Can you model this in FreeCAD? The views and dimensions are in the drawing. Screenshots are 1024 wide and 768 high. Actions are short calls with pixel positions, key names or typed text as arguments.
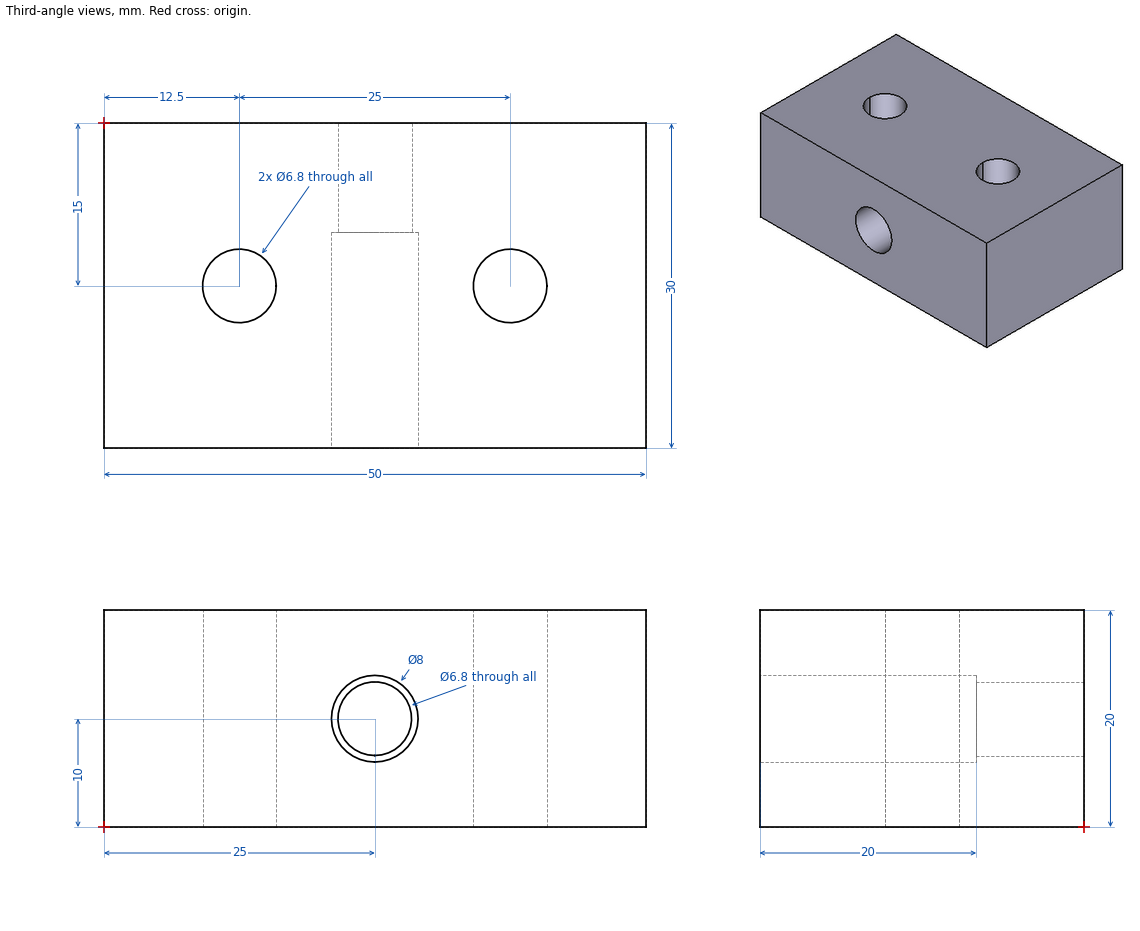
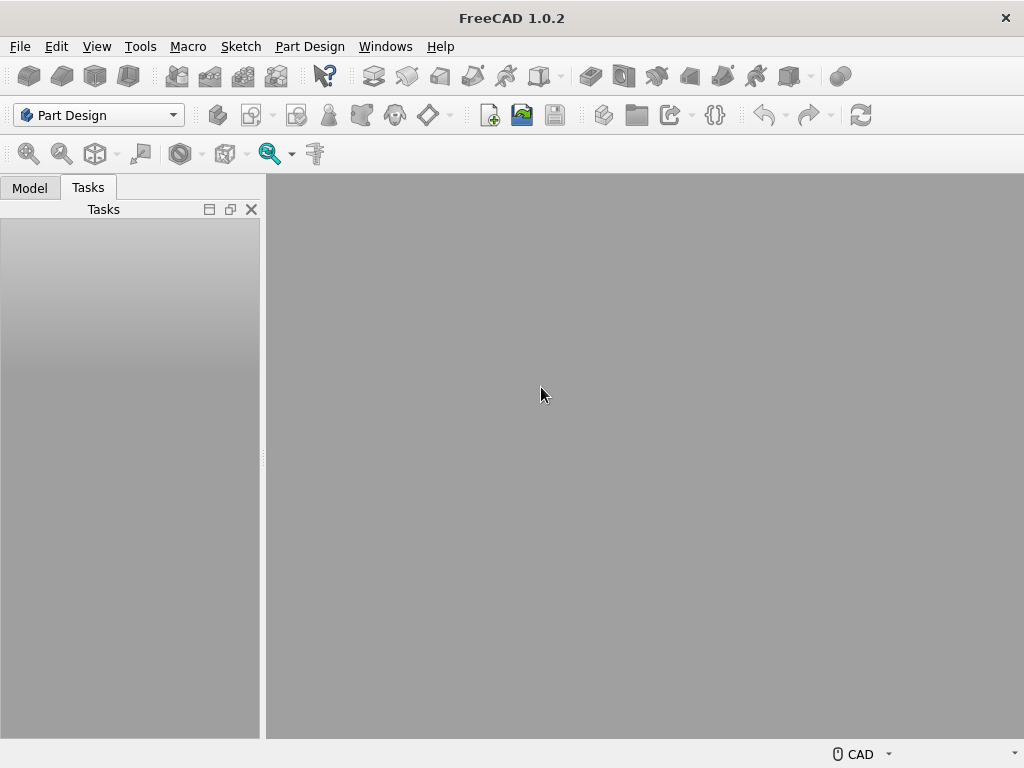
click(489, 116)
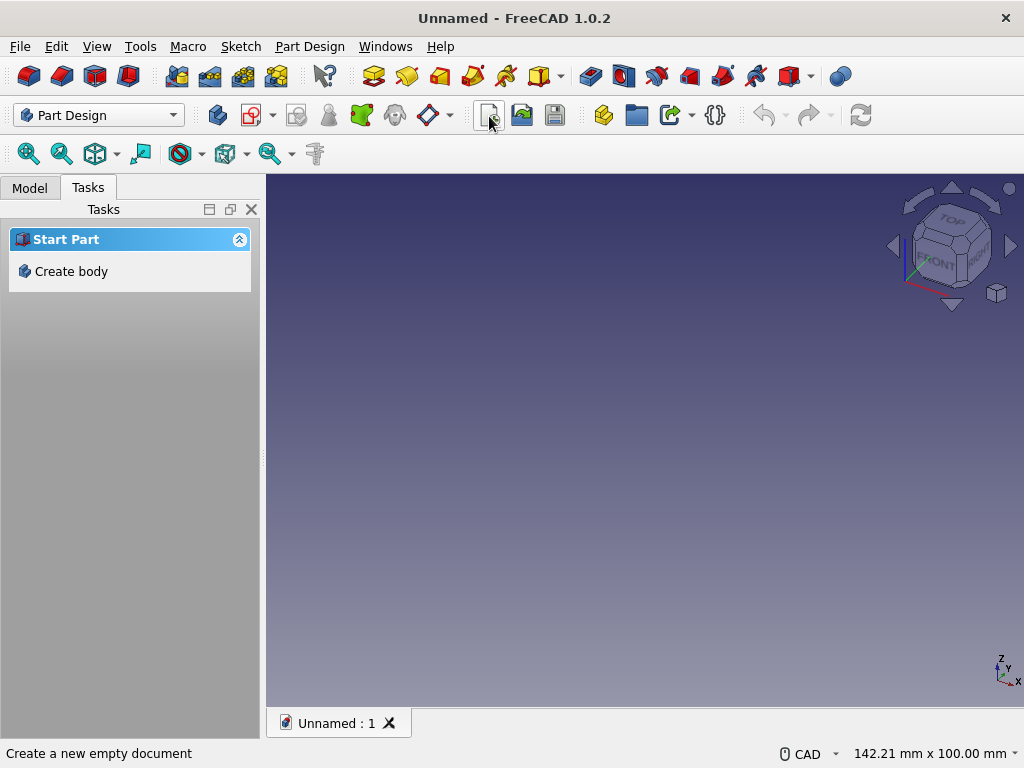
click(250, 116)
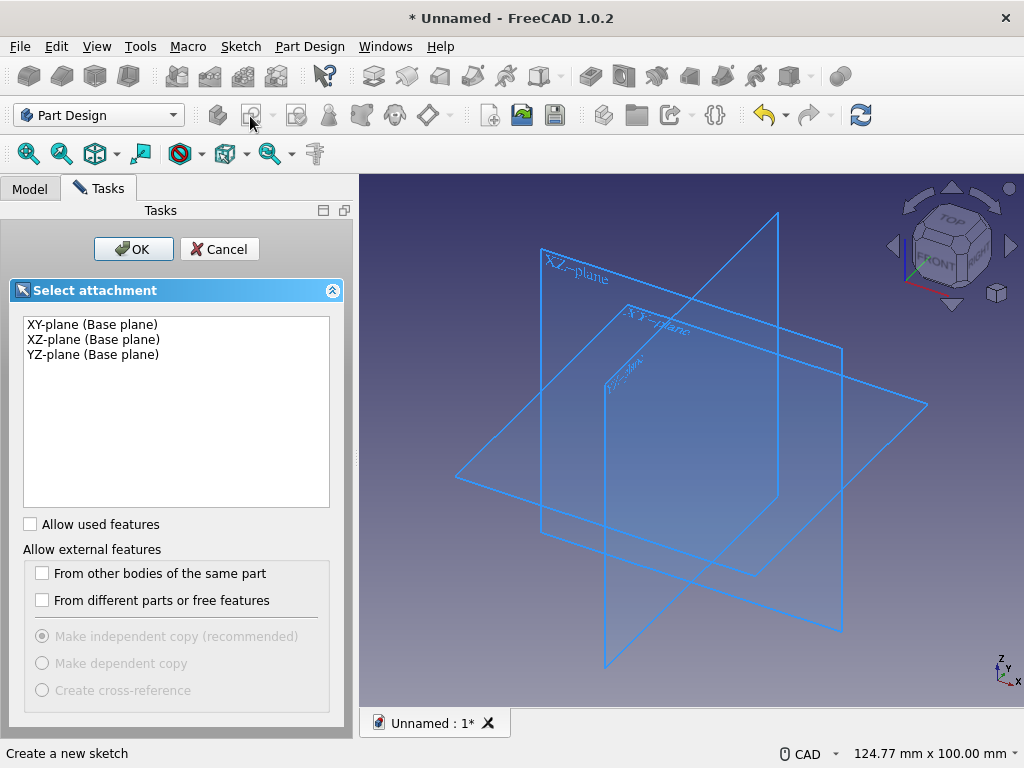
click(84, 324)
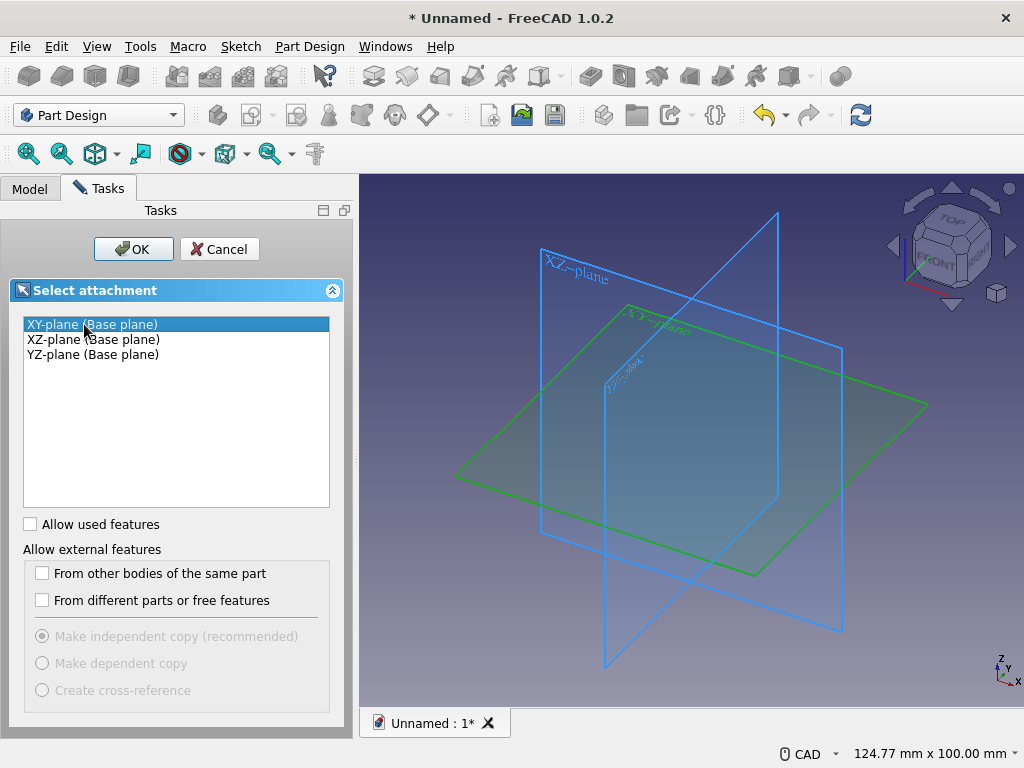
click(134, 249)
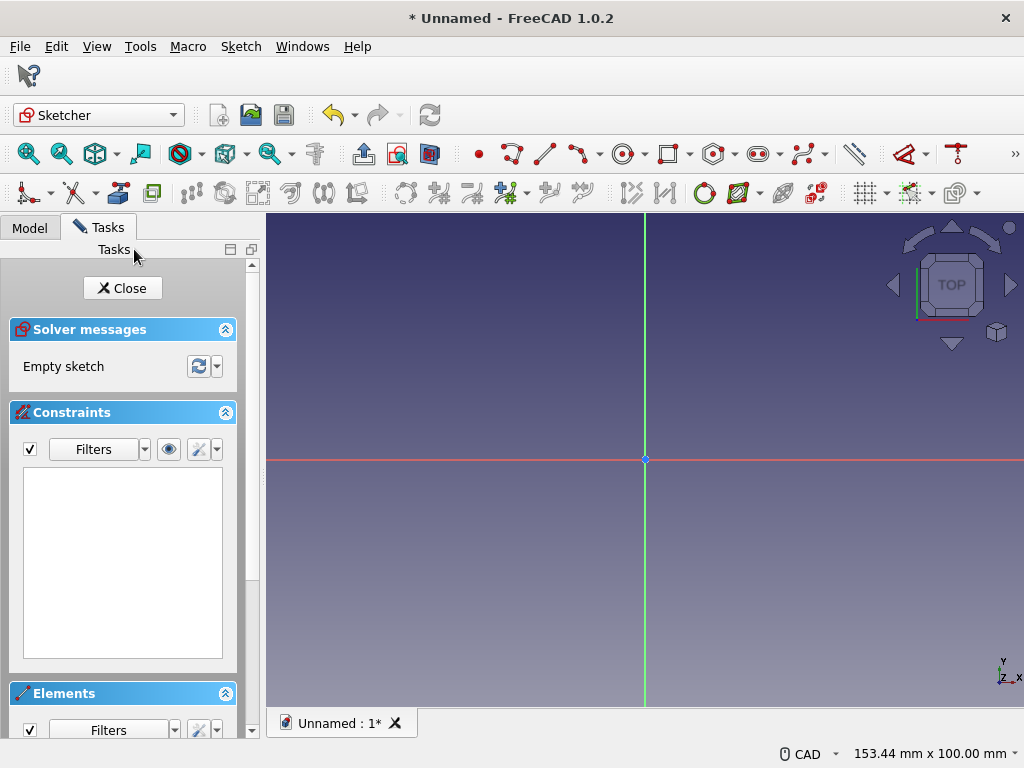
scroll(294, 241, down, 1)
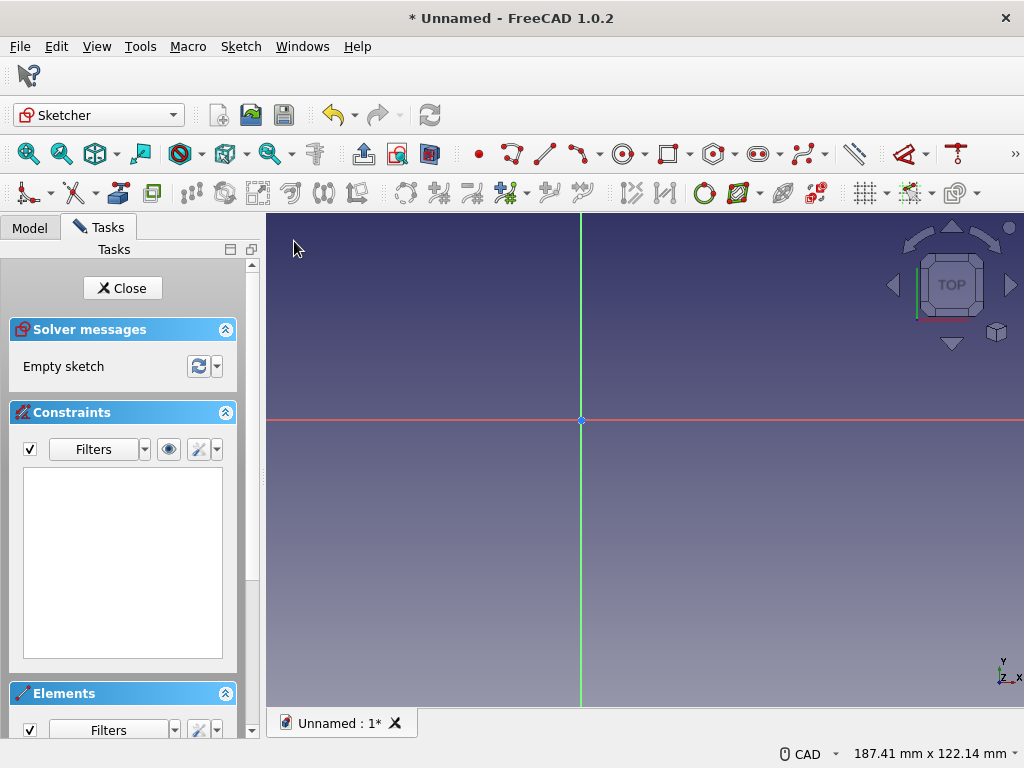
scroll(811, 507, up, 3)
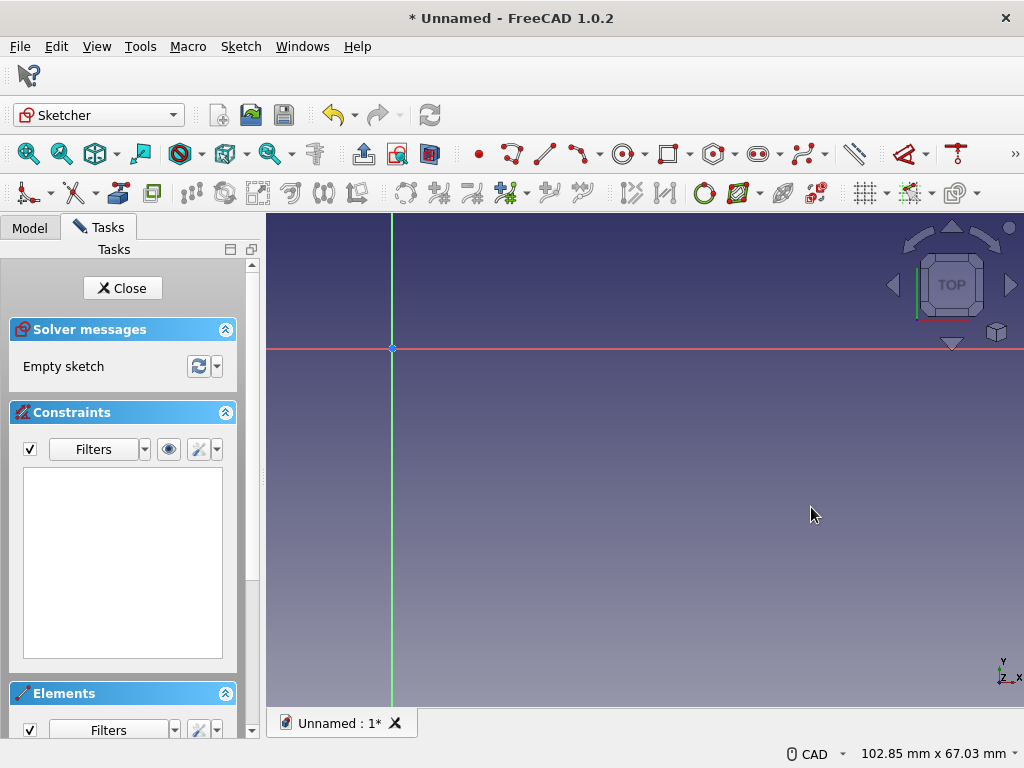
click(668, 154)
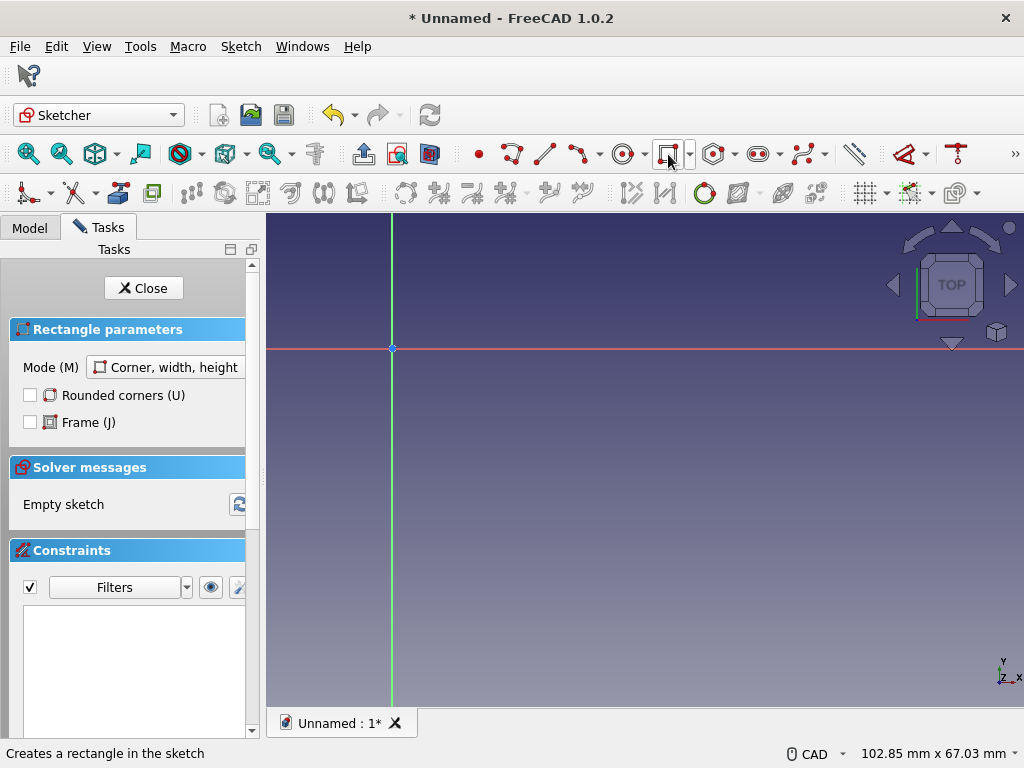
click(392, 349)
move(760, 570)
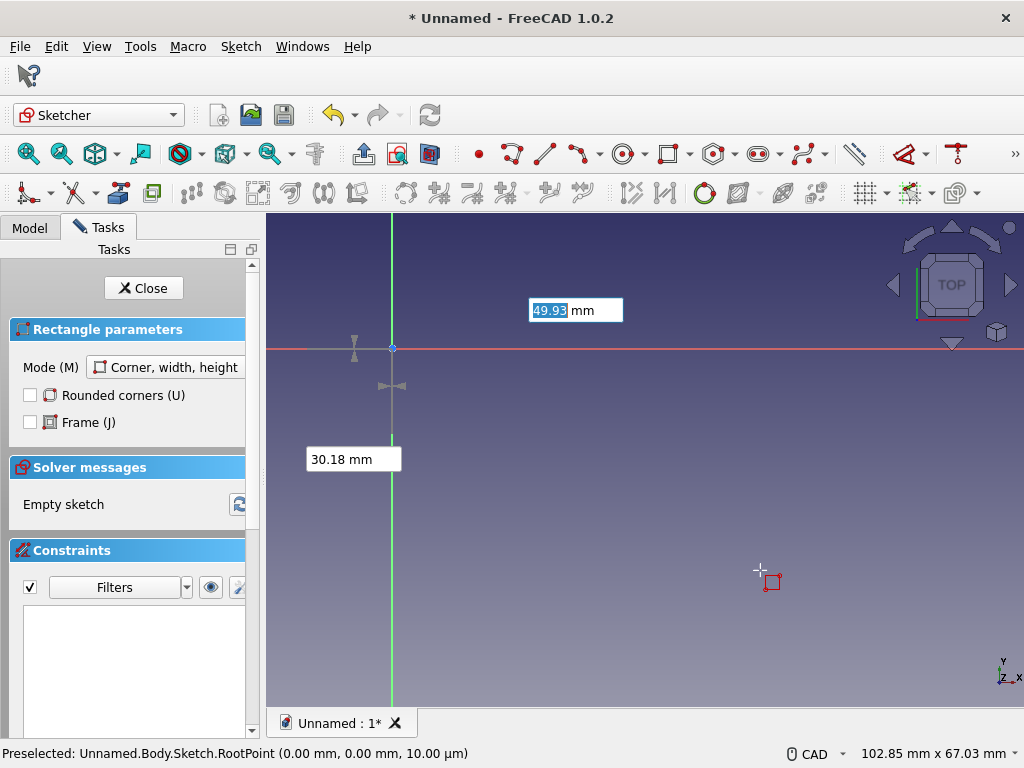
text(50)
key(Tab)
text(30)
key(Return)
key(Escape)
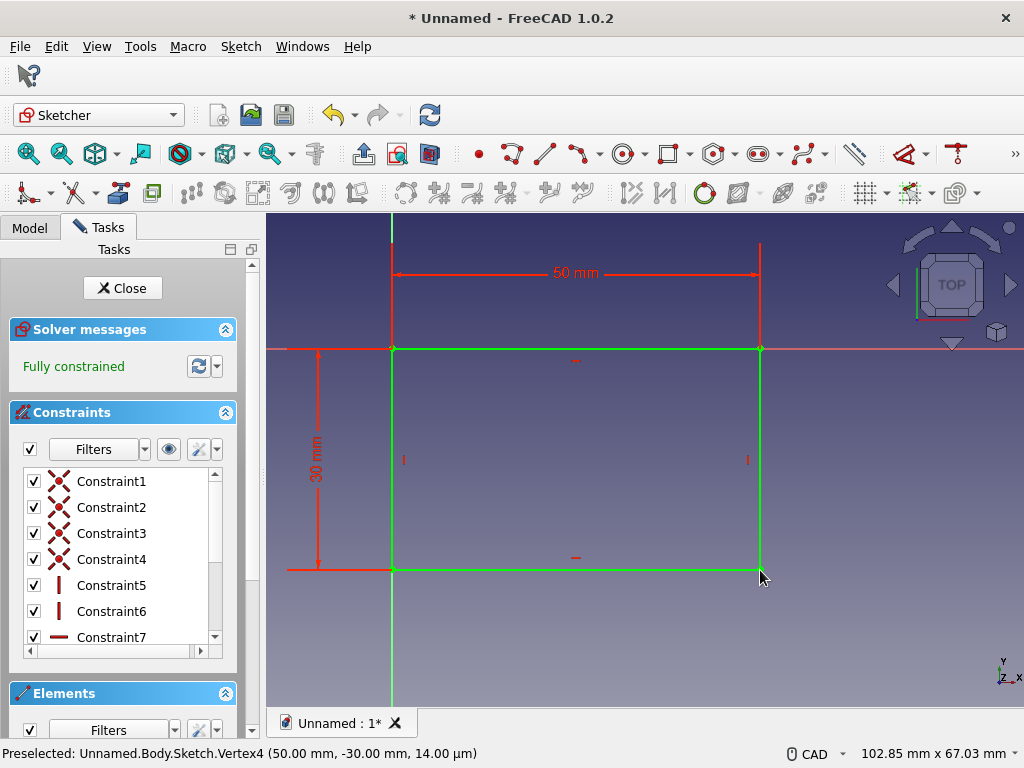
click(123, 288)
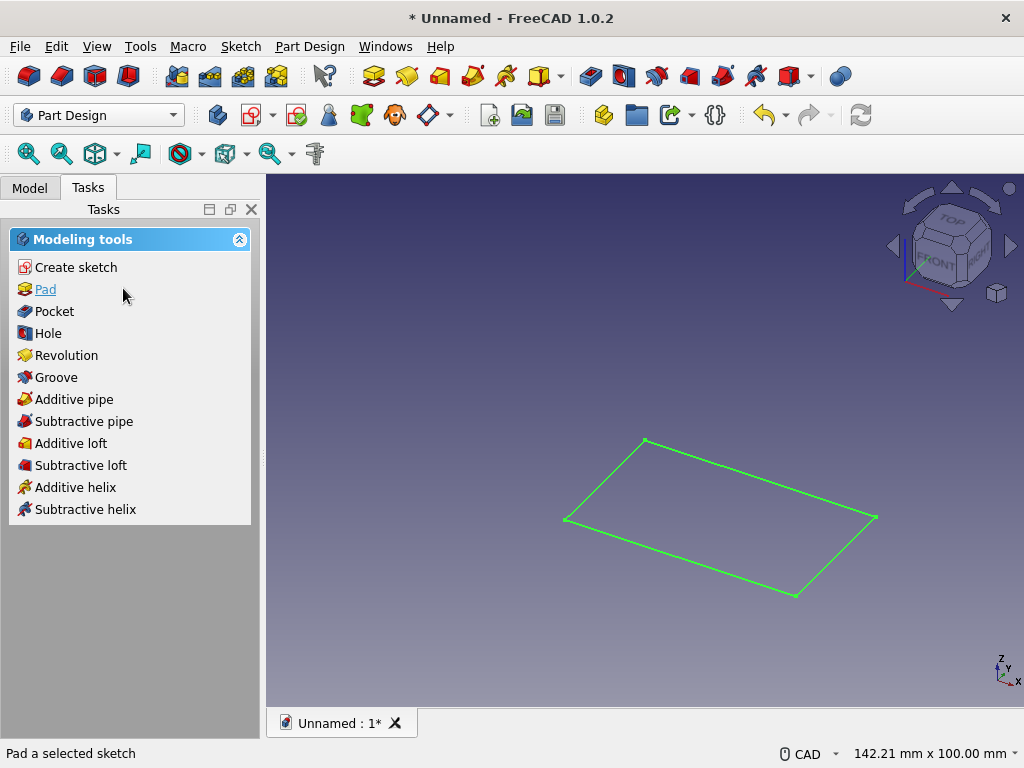
click(374, 76)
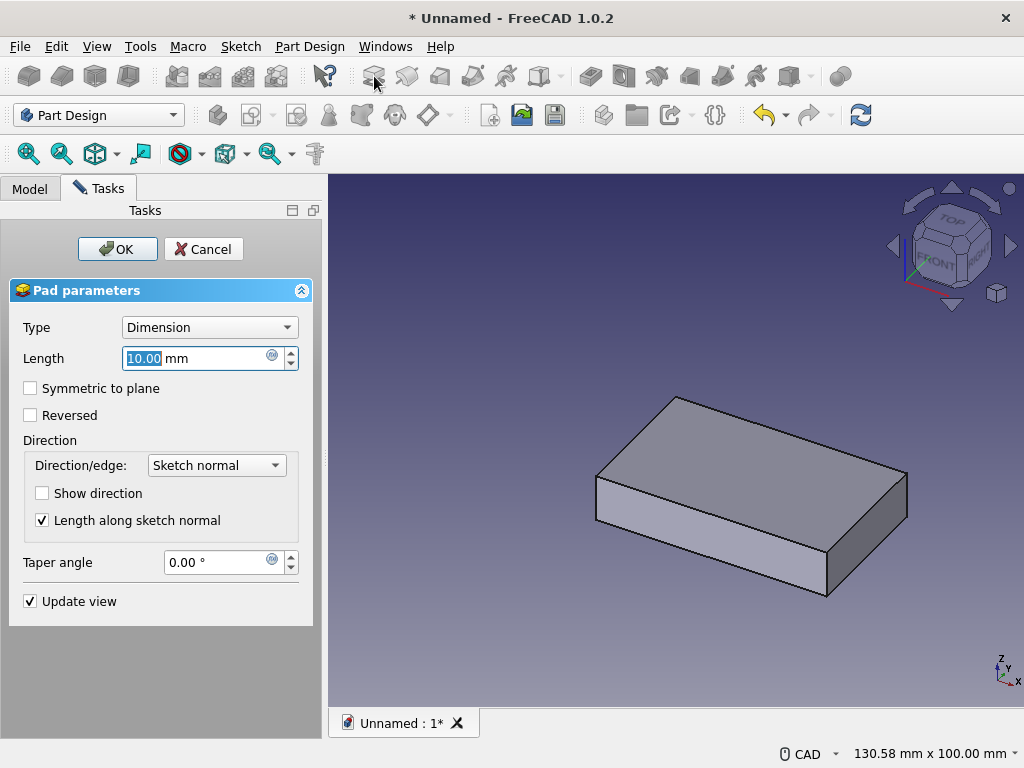
text(20)
key(Tab)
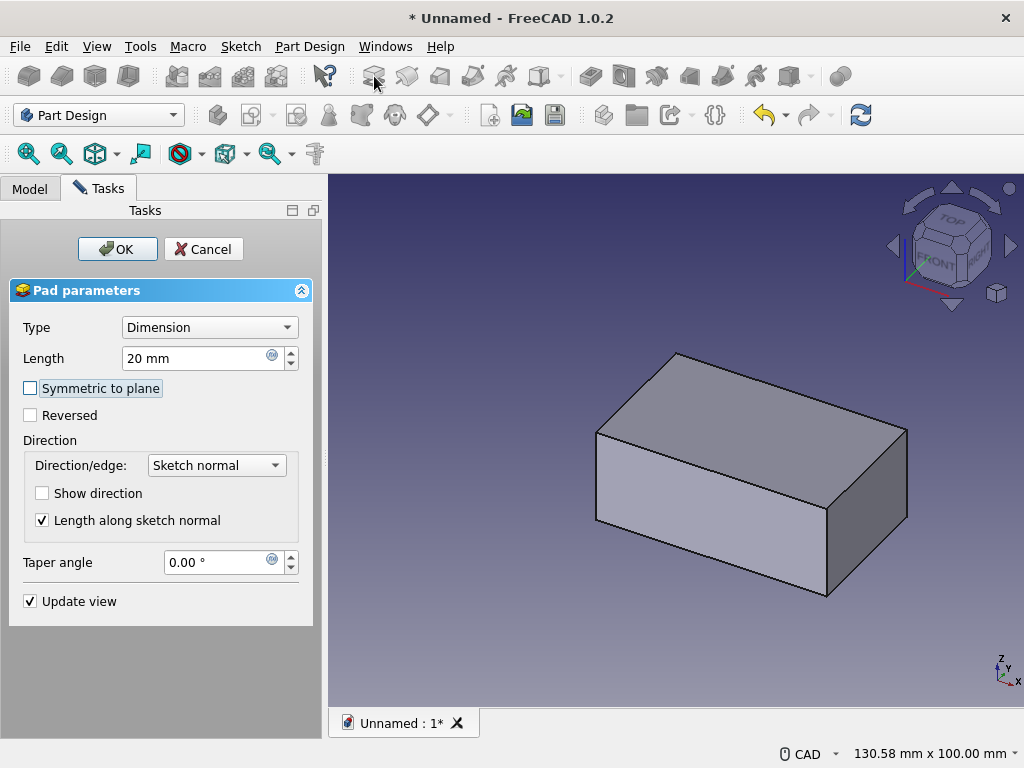
click(118, 249)